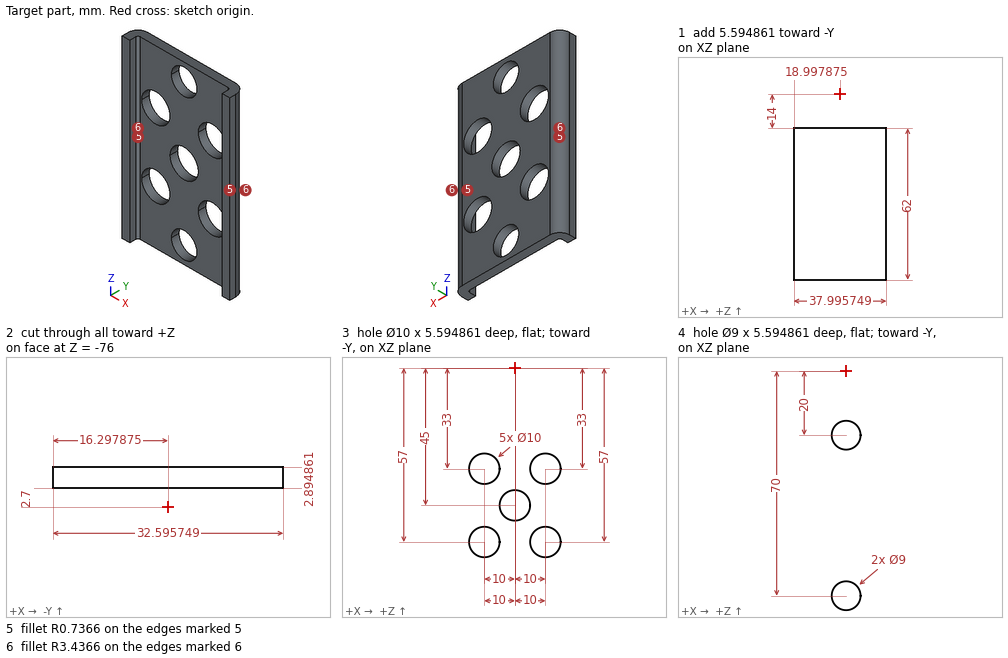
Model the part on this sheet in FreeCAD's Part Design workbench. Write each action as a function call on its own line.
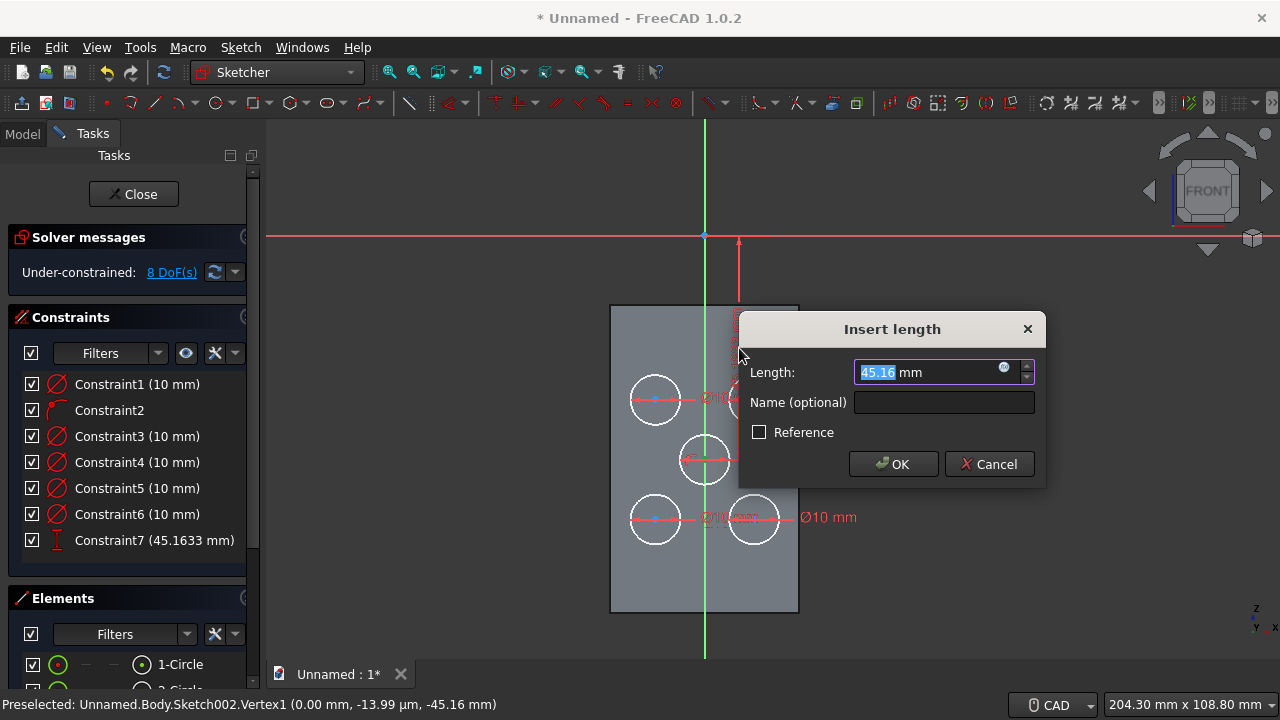
text(45)
key(Return)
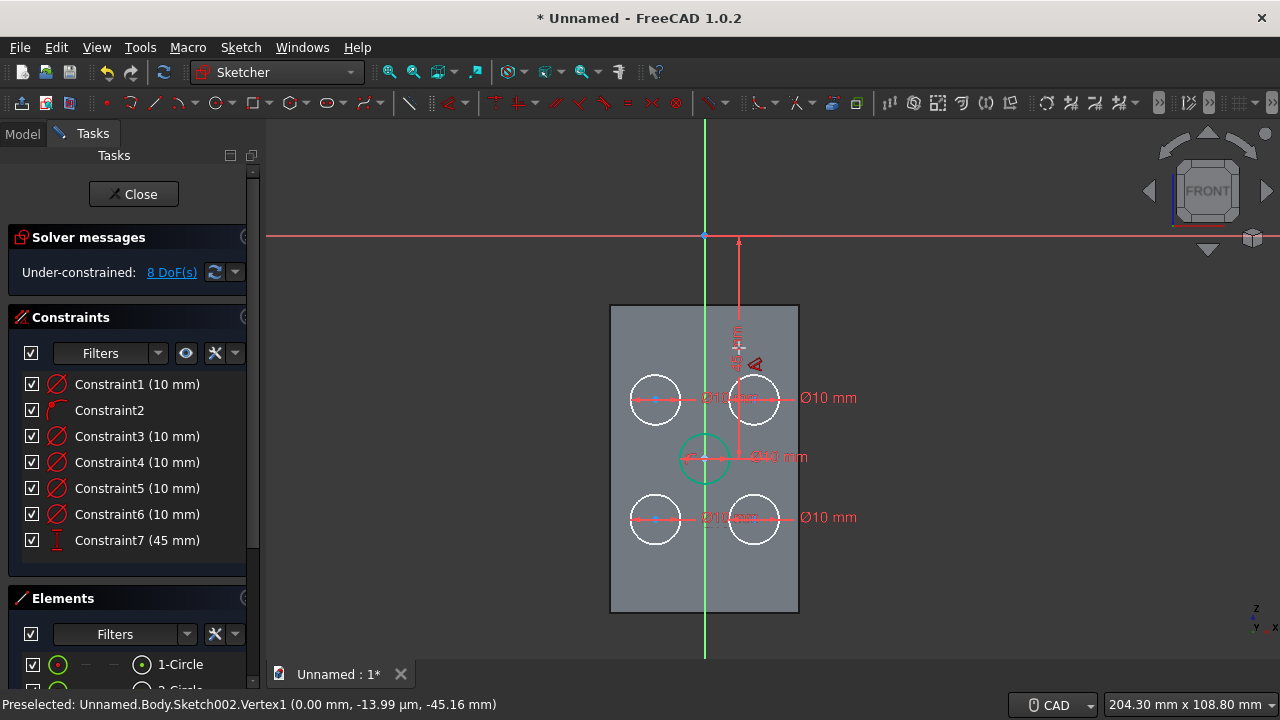
click(655, 520)
click(680, 202)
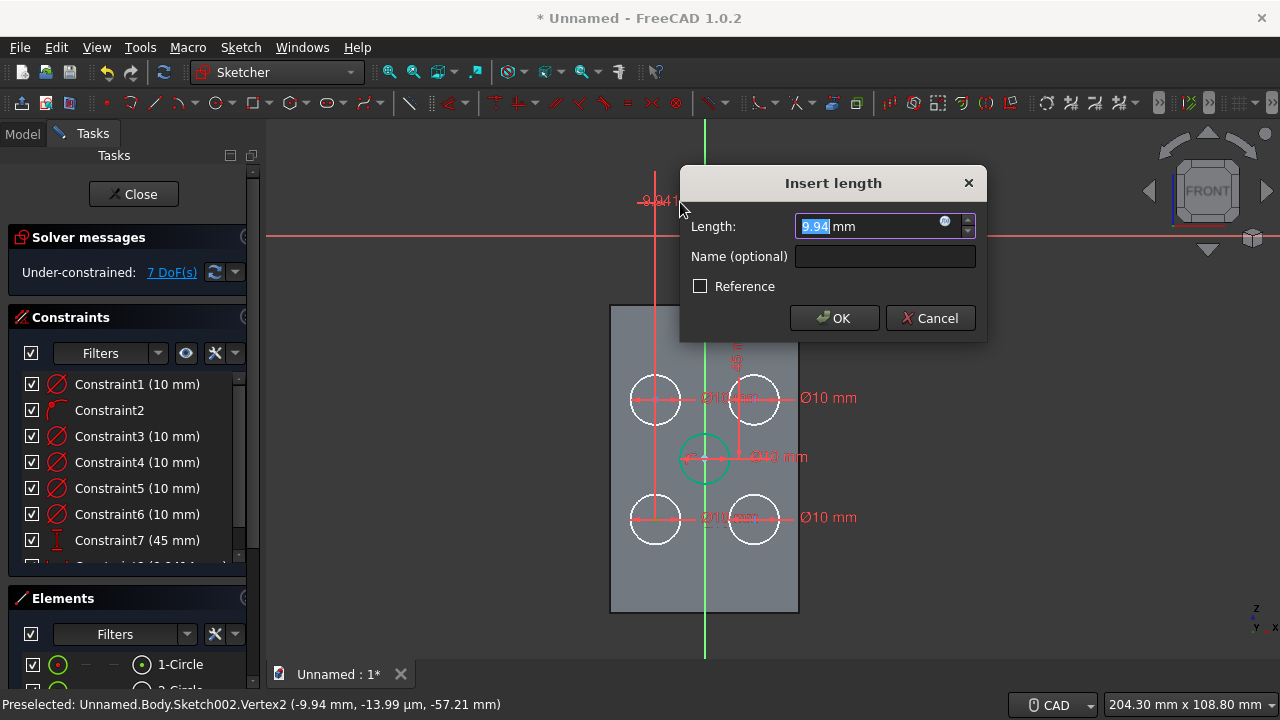
text(10)
key(Return)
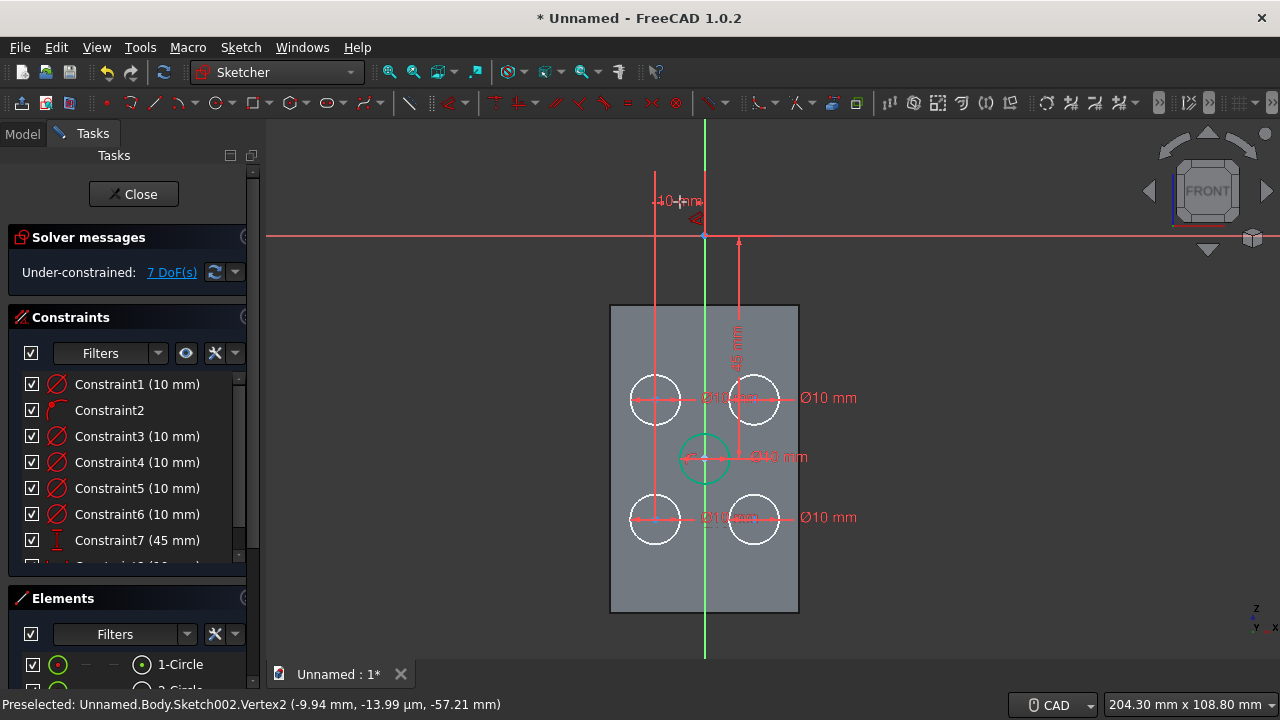
click(655, 520)
click(621, 378)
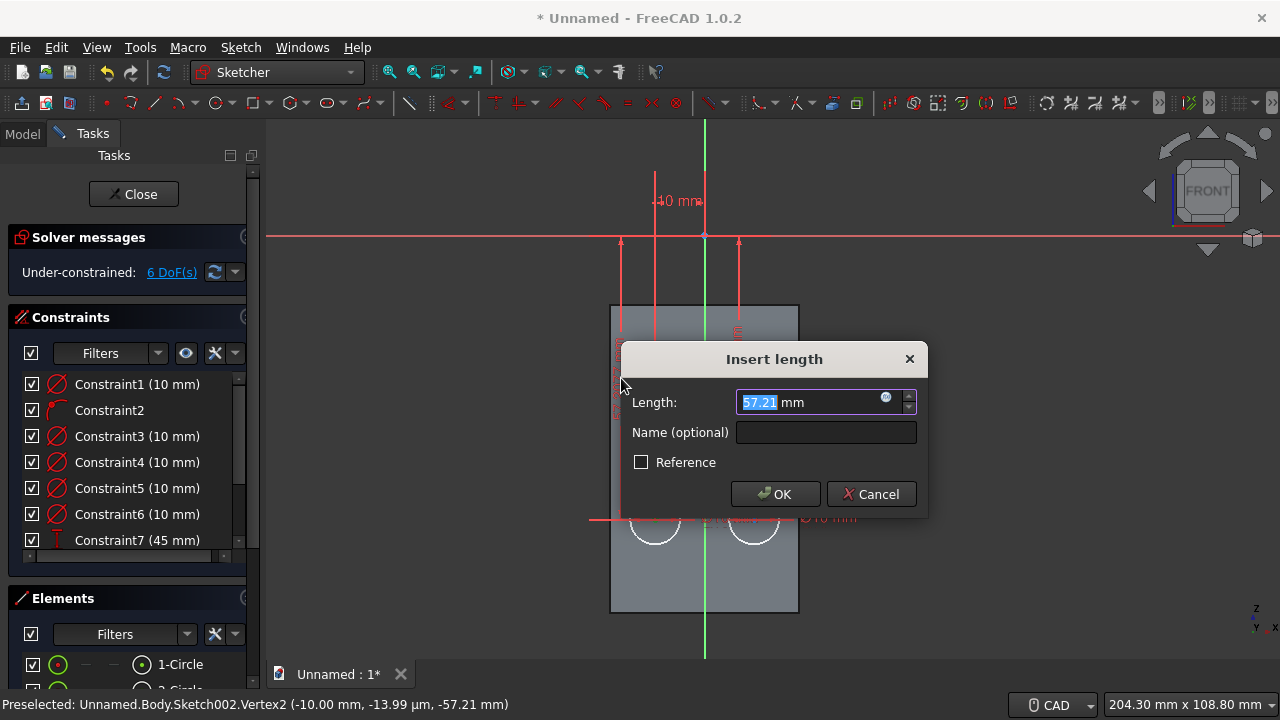
text(57)
key(Return)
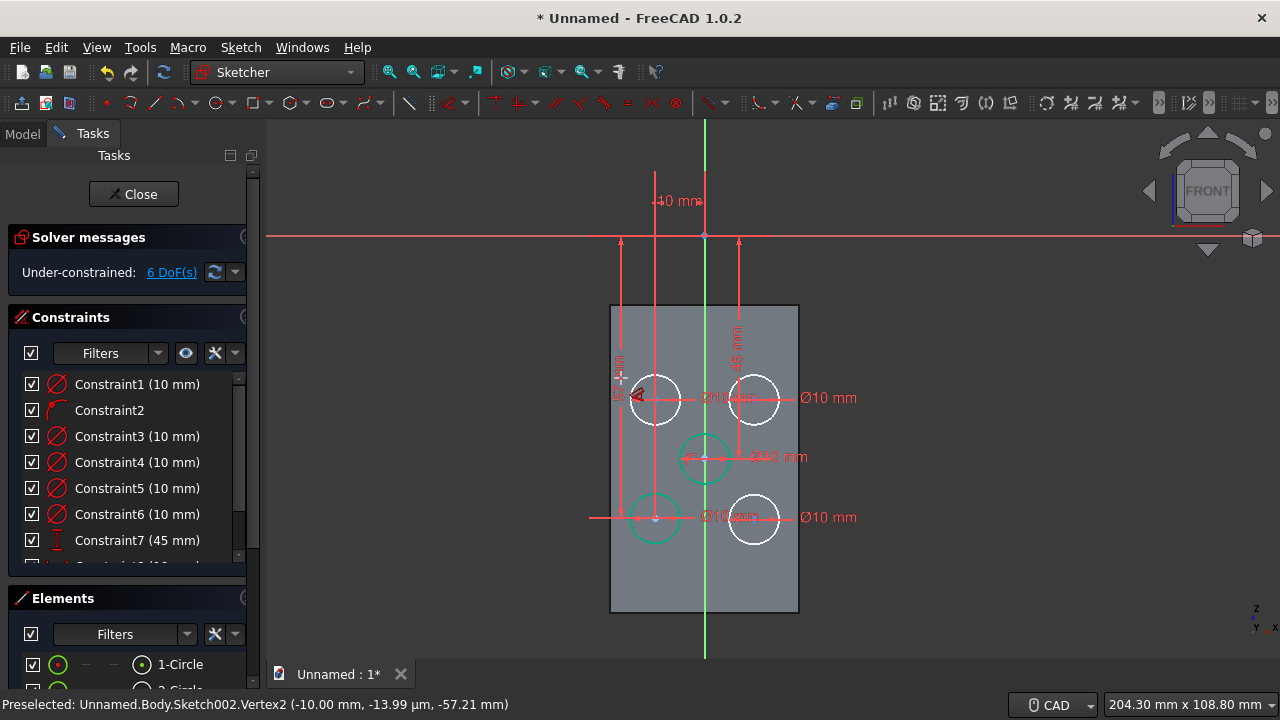
click(655, 400)
click(680, 178)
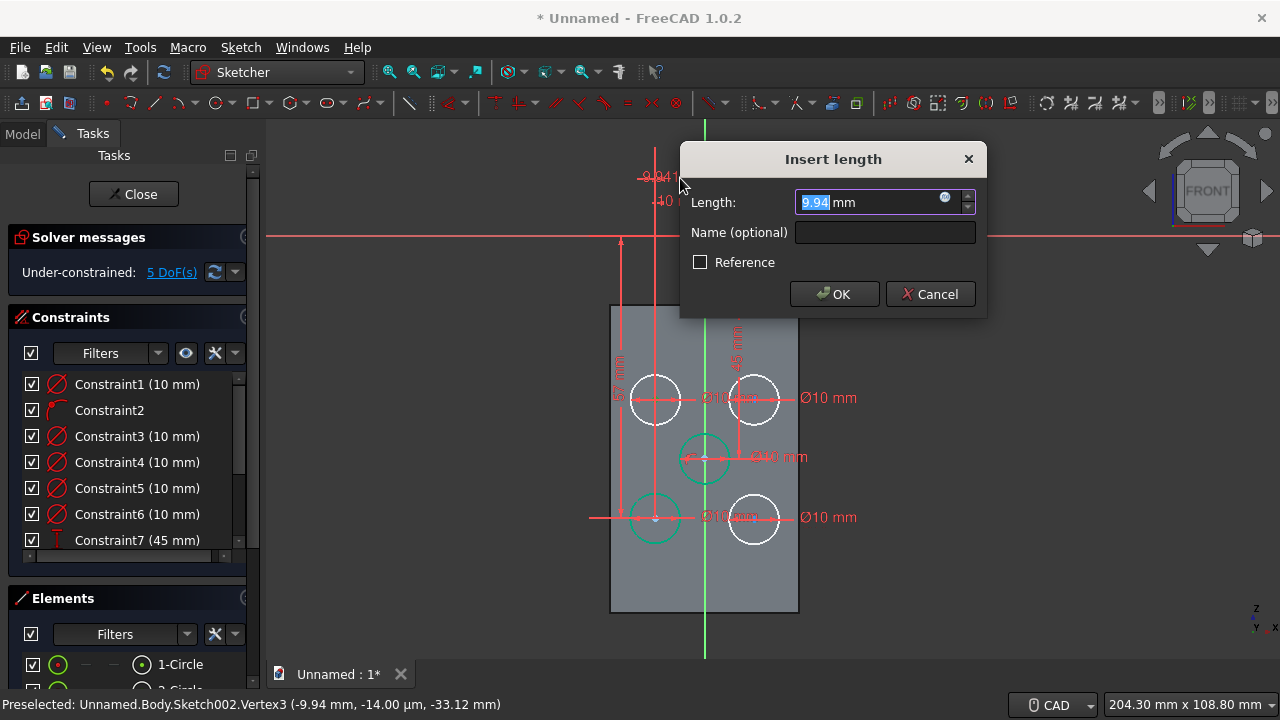
text(10)
key(Return)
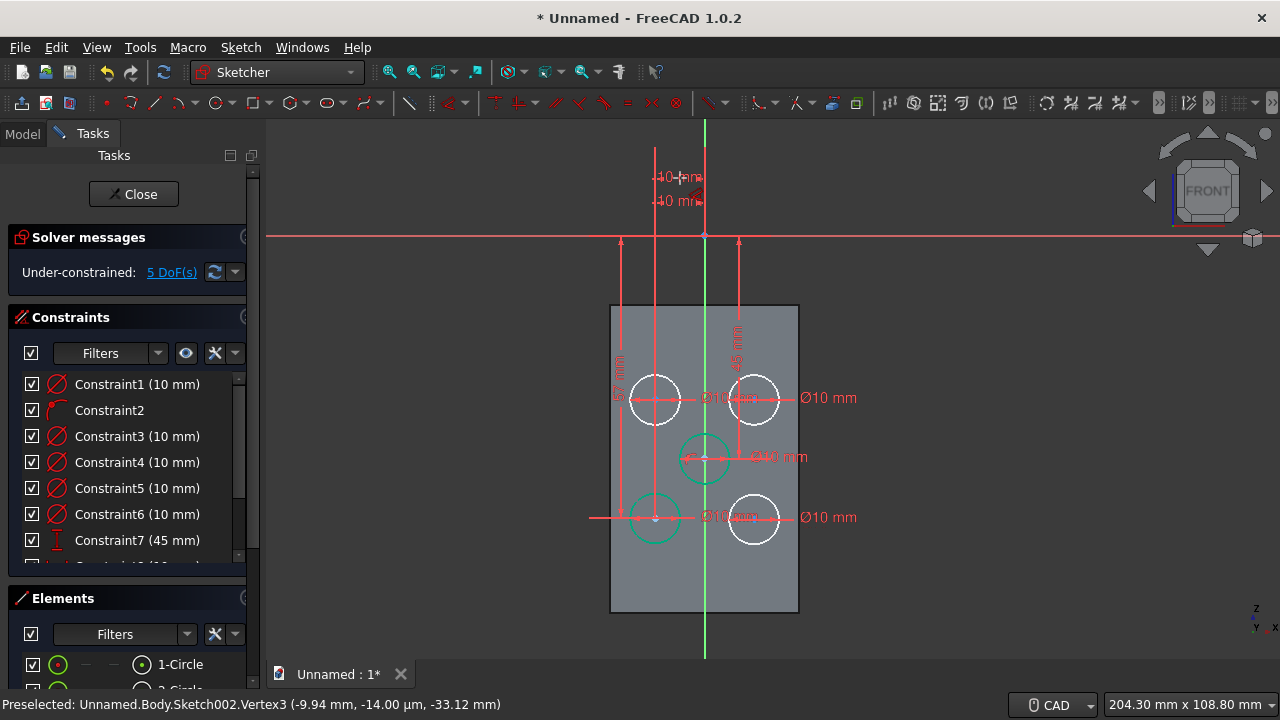
click(655, 400)
click(621, 318)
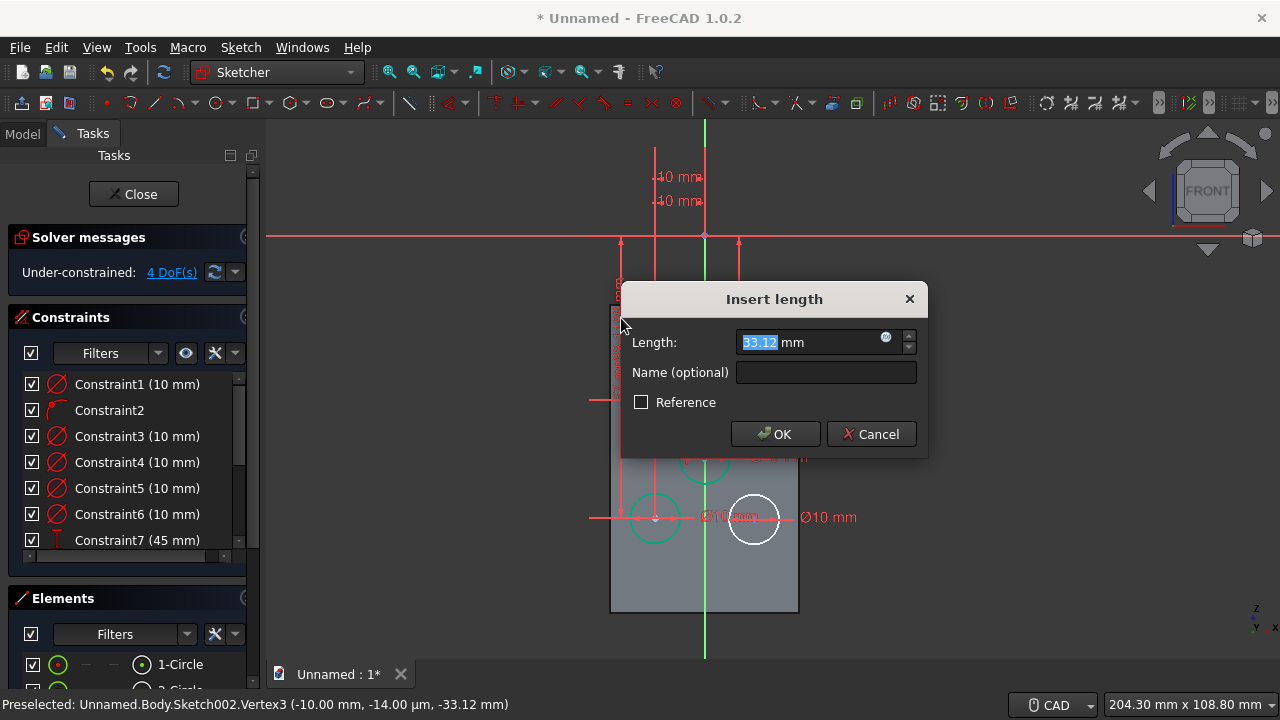
text(33)
key(Return)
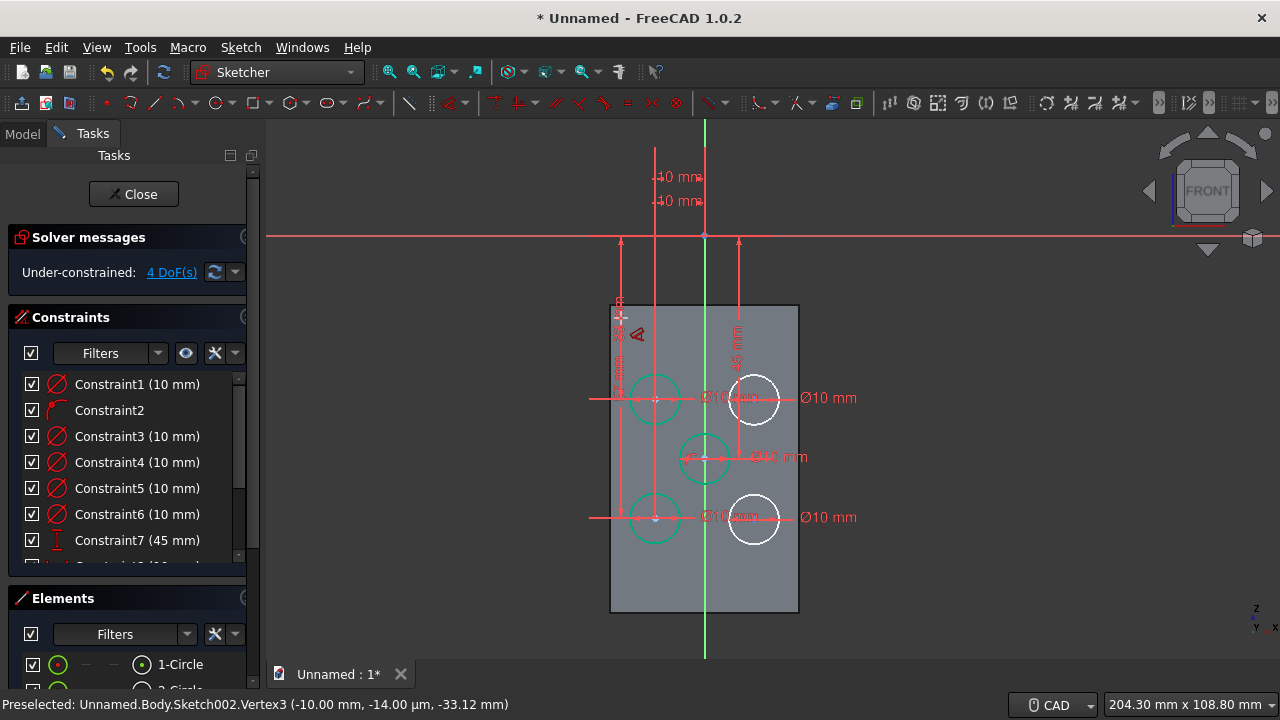
click(754, 400)
click(747, 458)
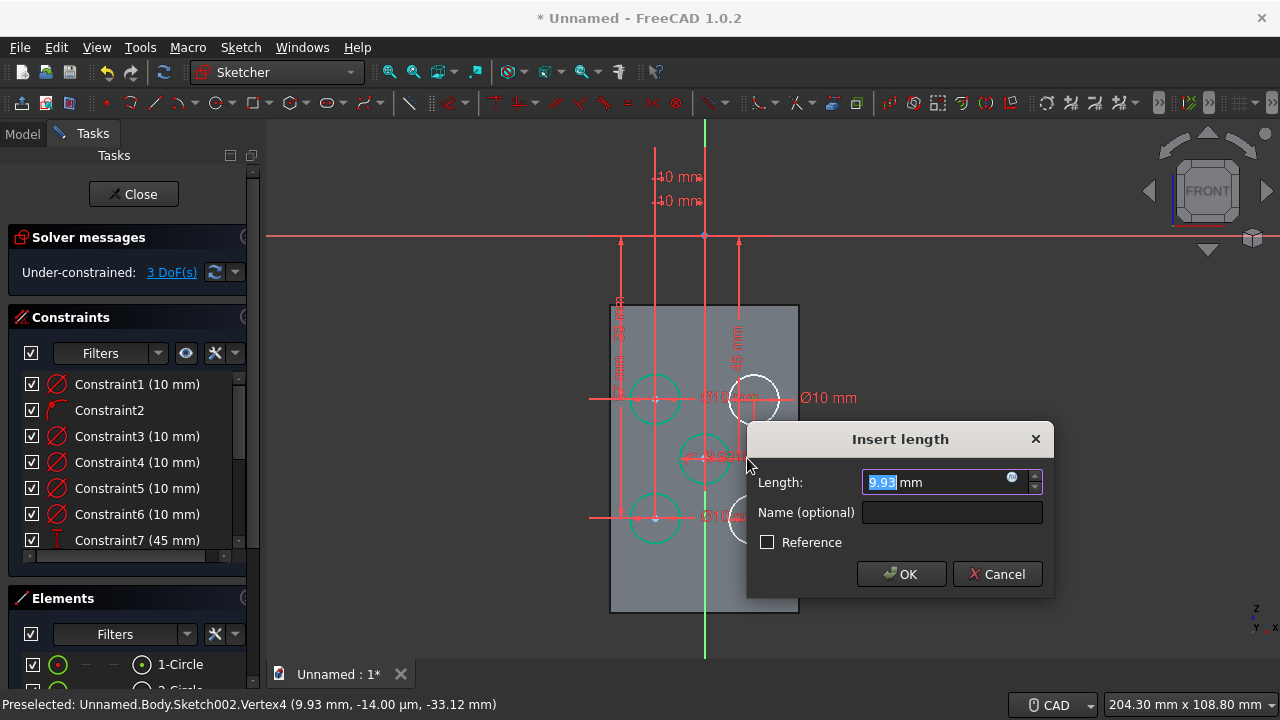
text(10)
key(Return)